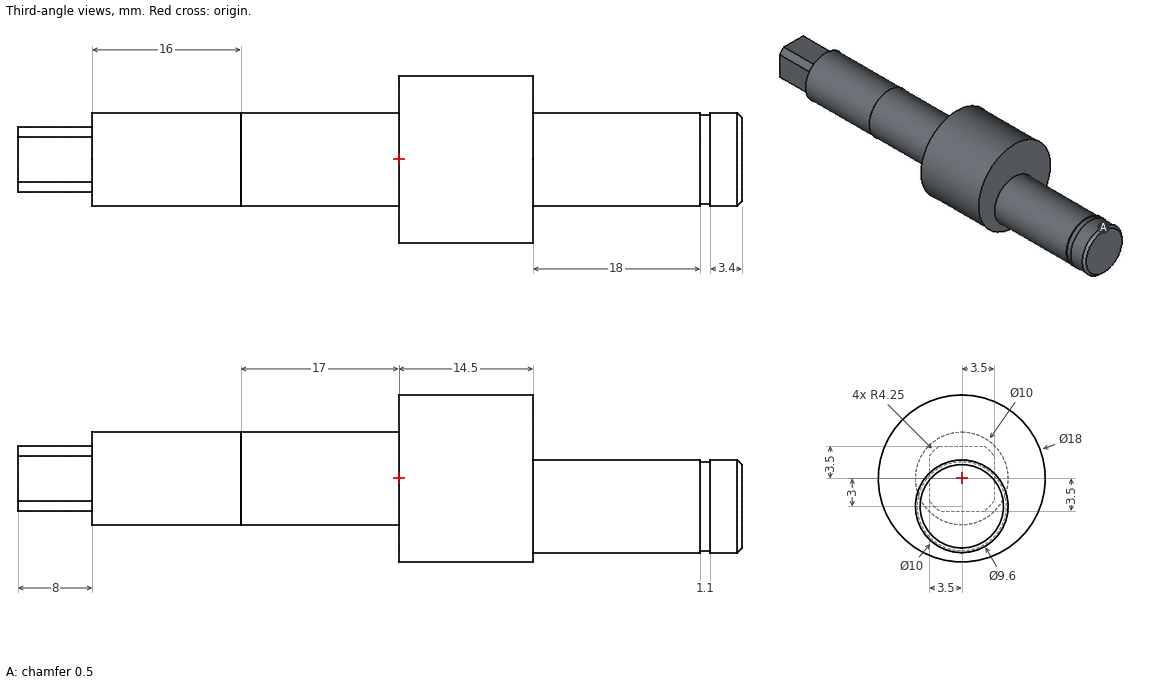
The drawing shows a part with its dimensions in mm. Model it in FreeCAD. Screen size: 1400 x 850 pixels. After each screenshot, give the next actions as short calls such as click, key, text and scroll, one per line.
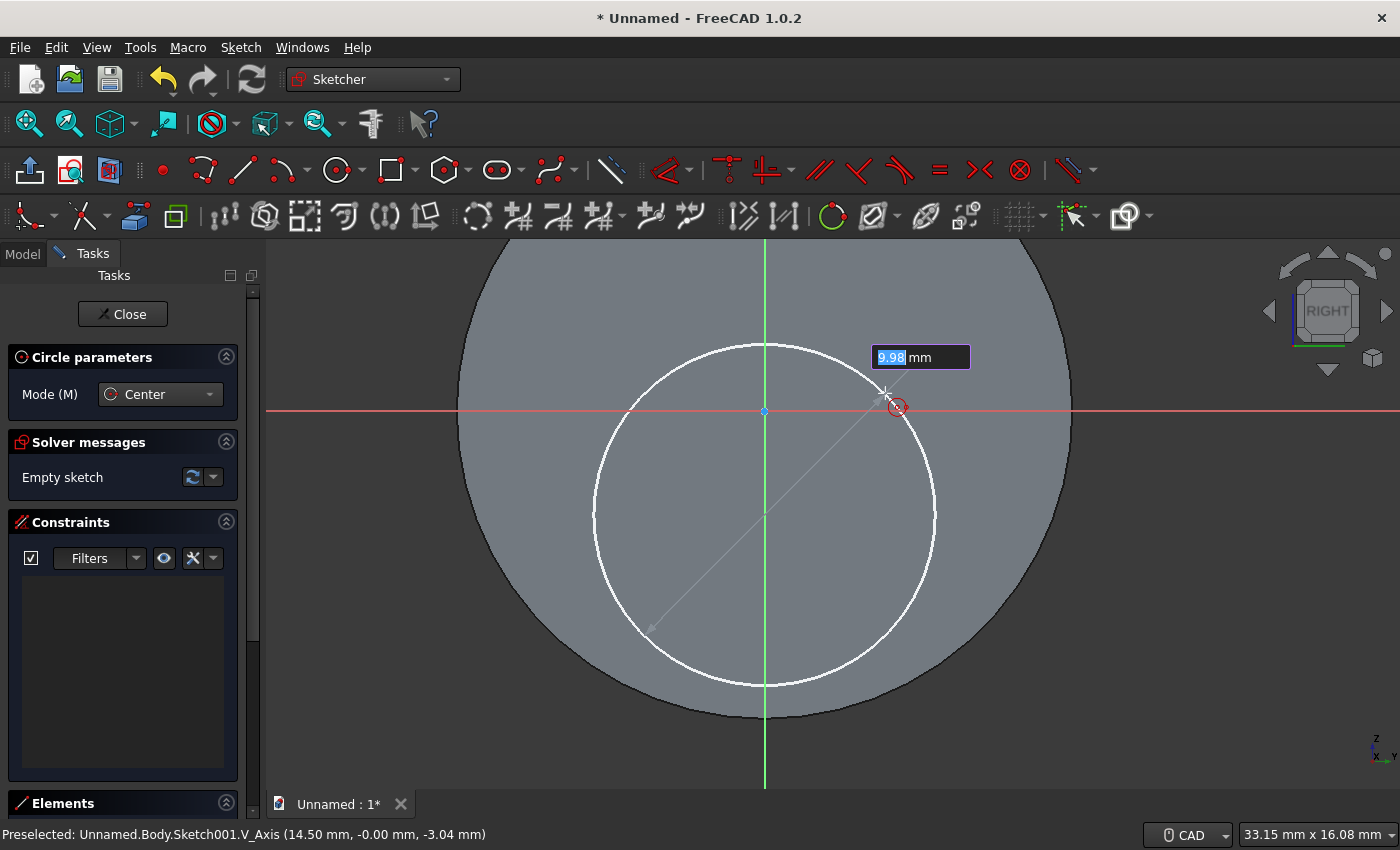
text(10)
key(Return)
key(Escape)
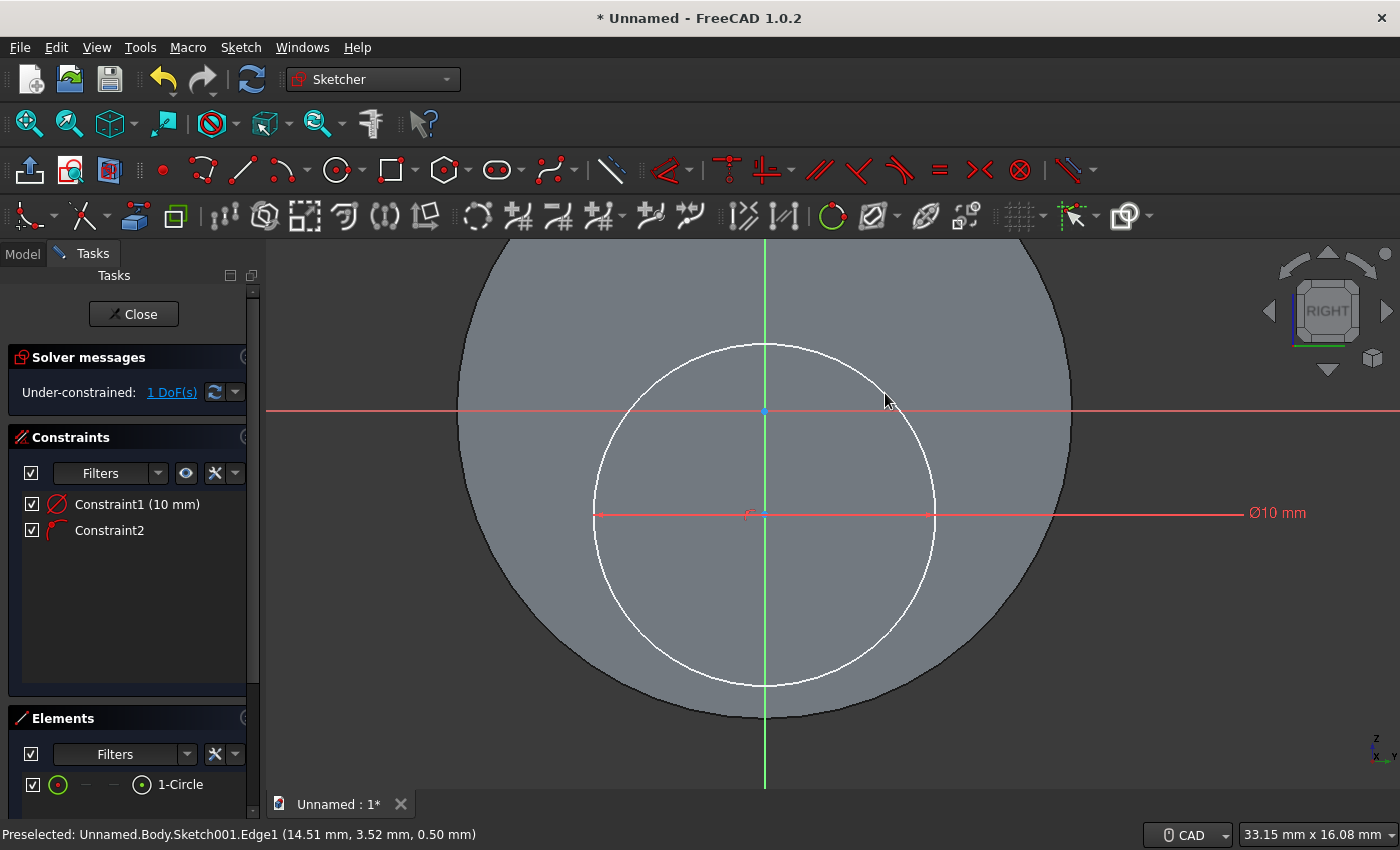
click(666, 170)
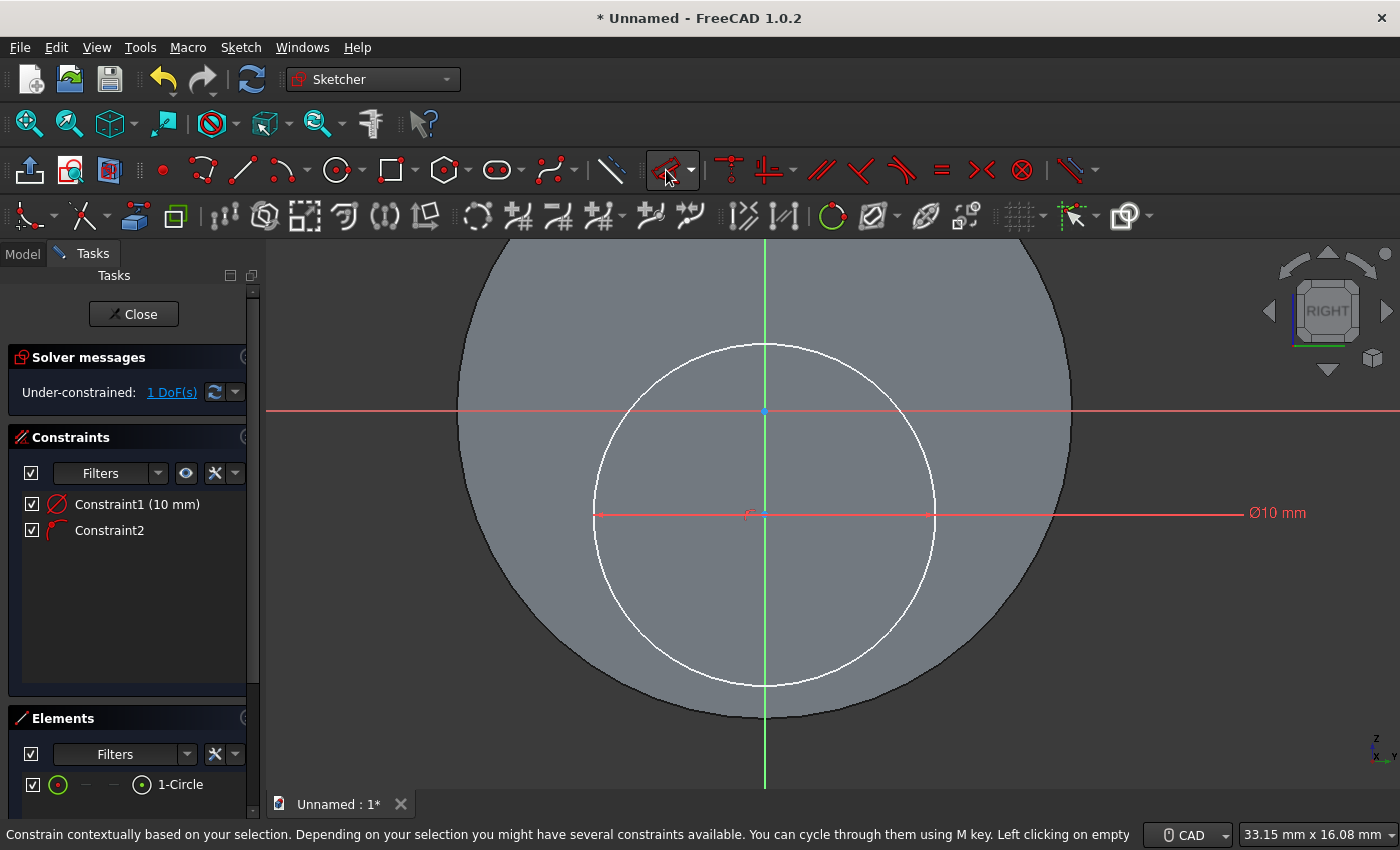
click(765, 515)
click(799, 463)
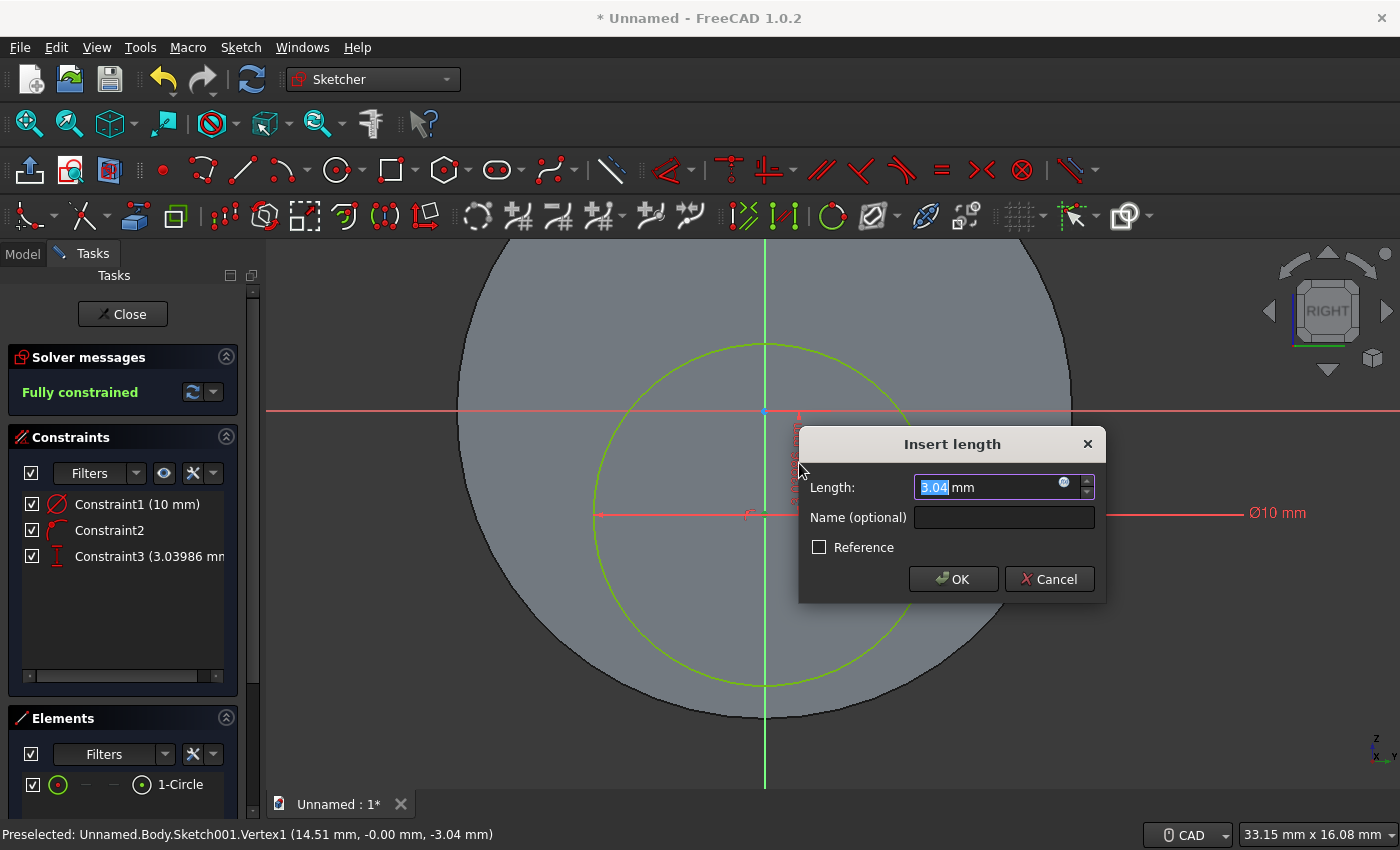
text(3)
key(Return)
key(Escape)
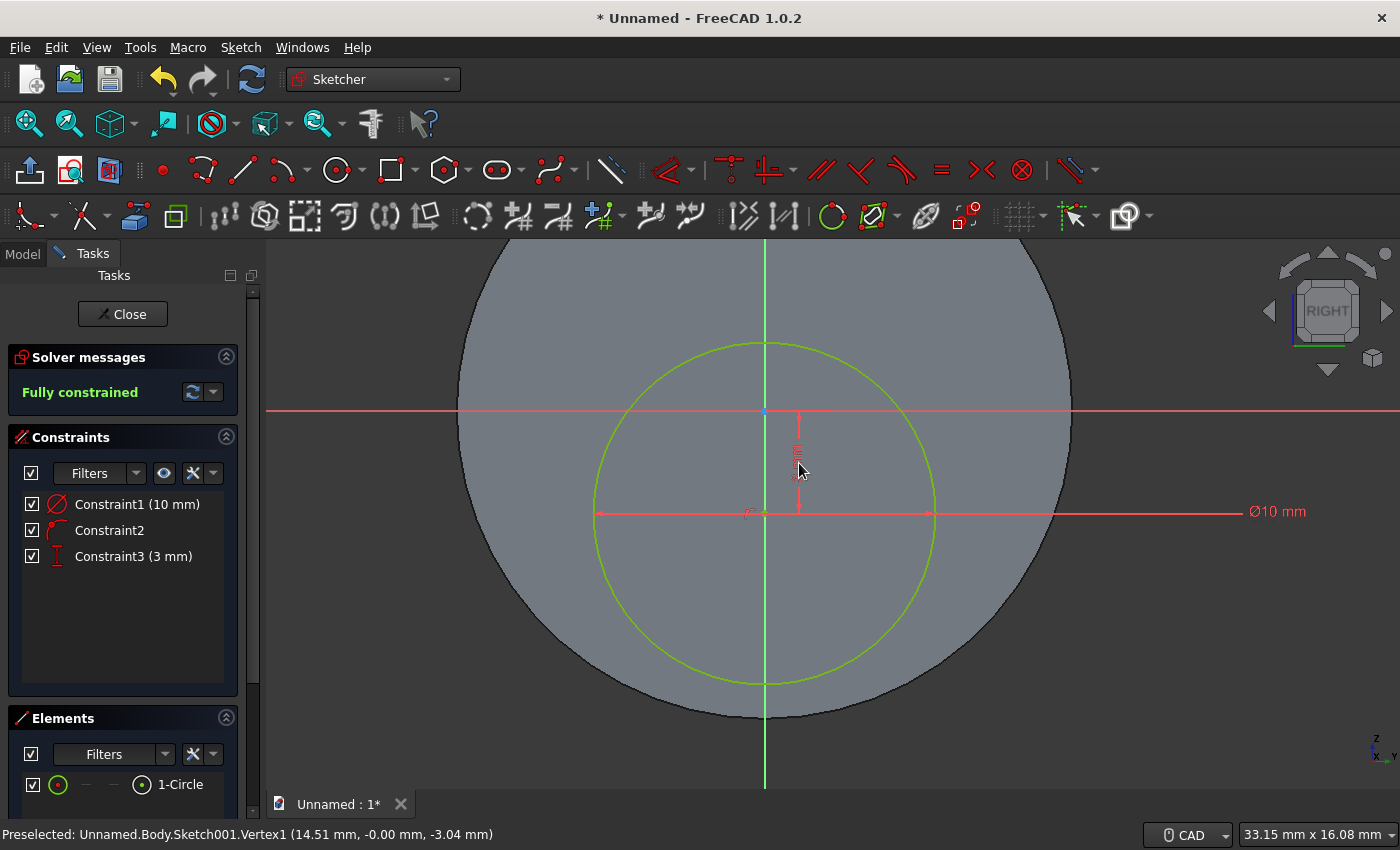
click(123, 314)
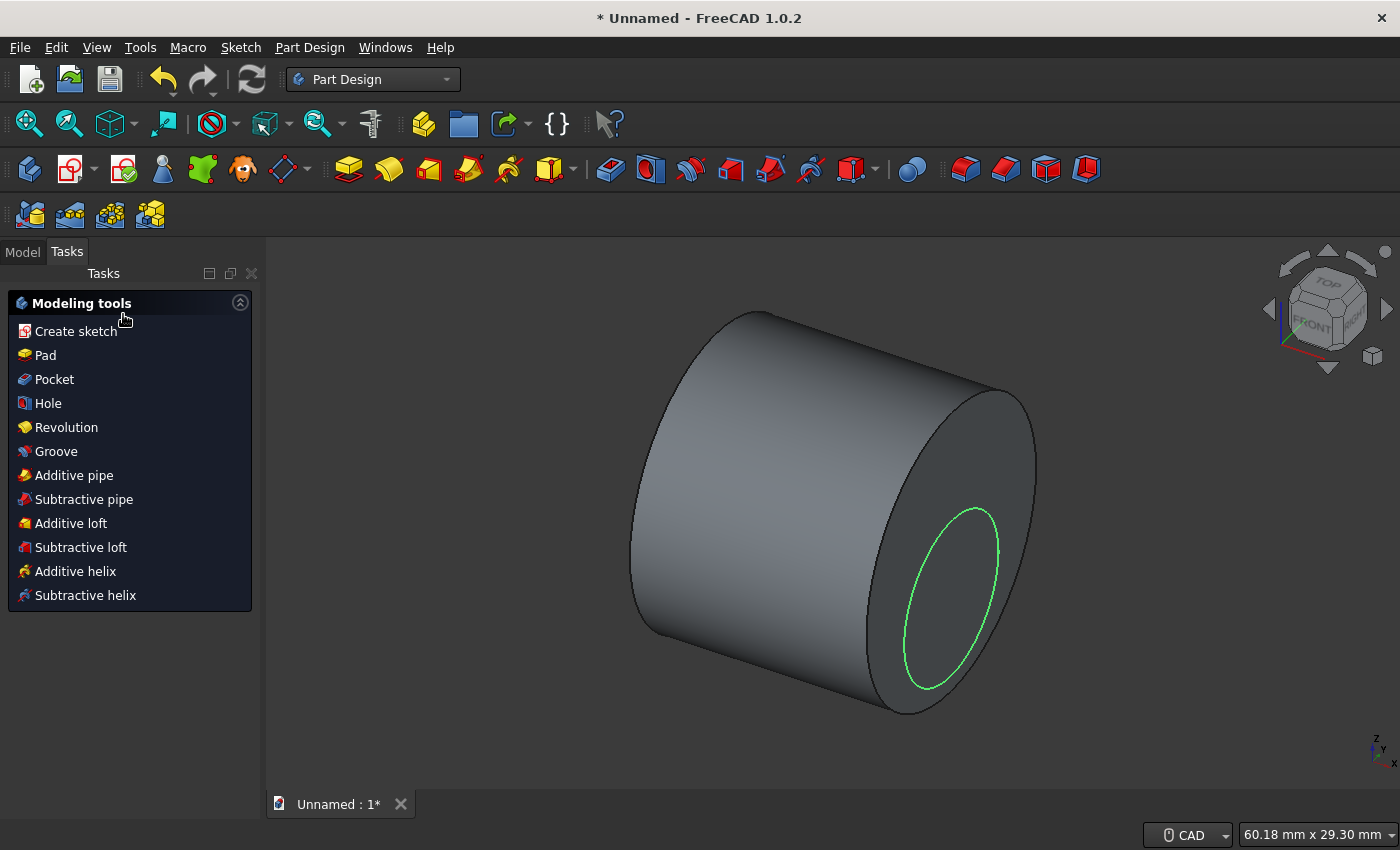
click(350, 170)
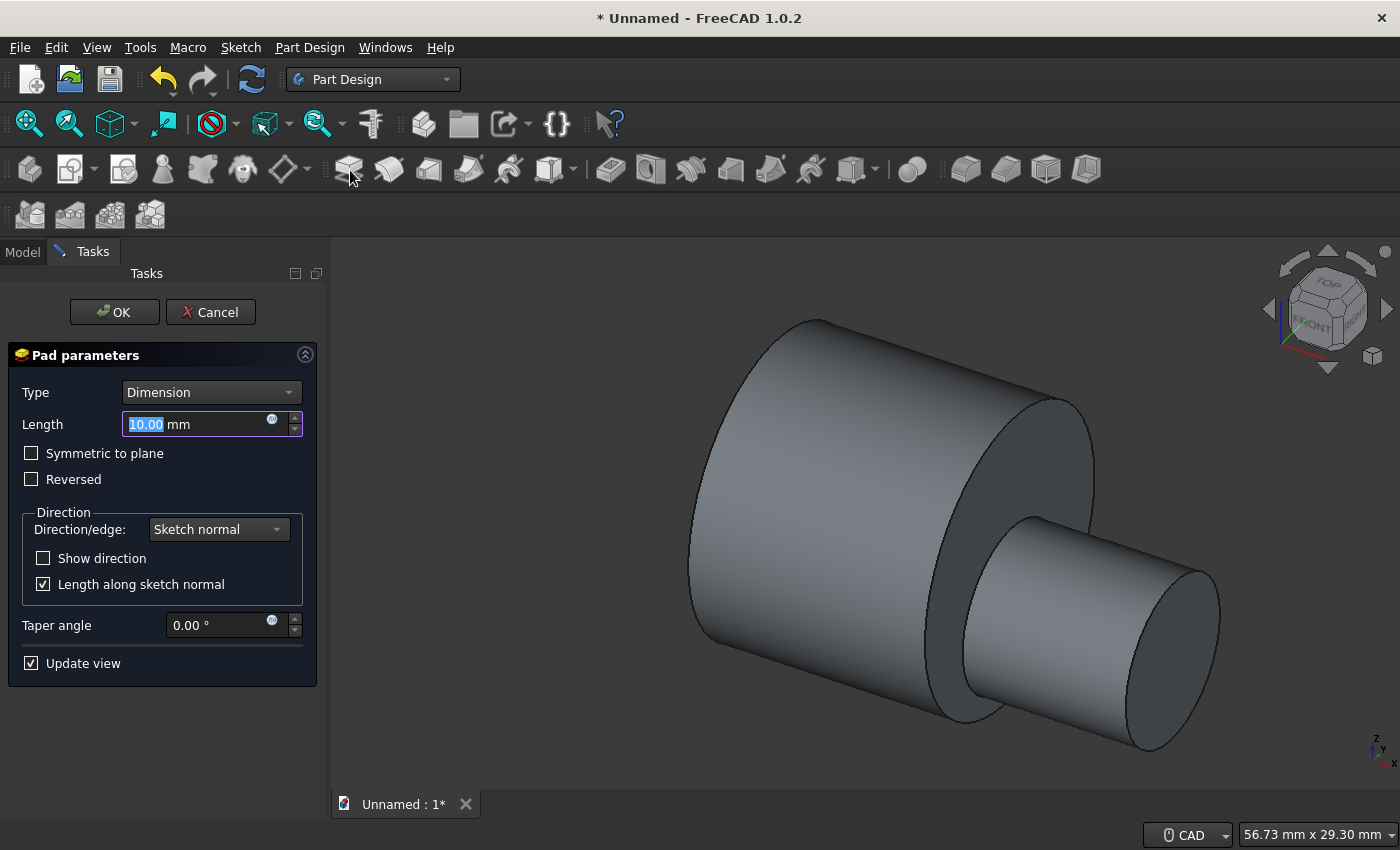
text(18)
key(Tab)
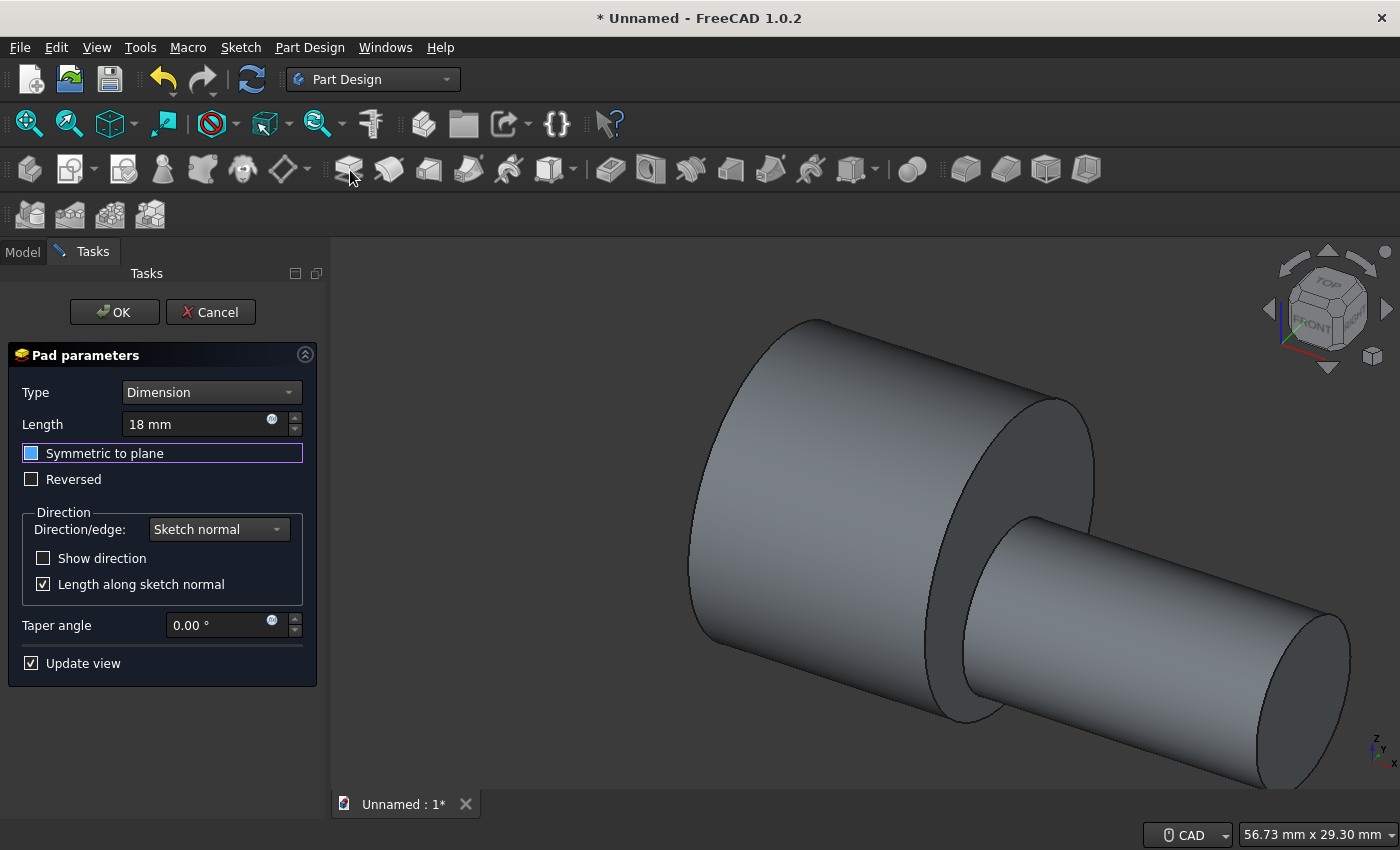
click(115, 312)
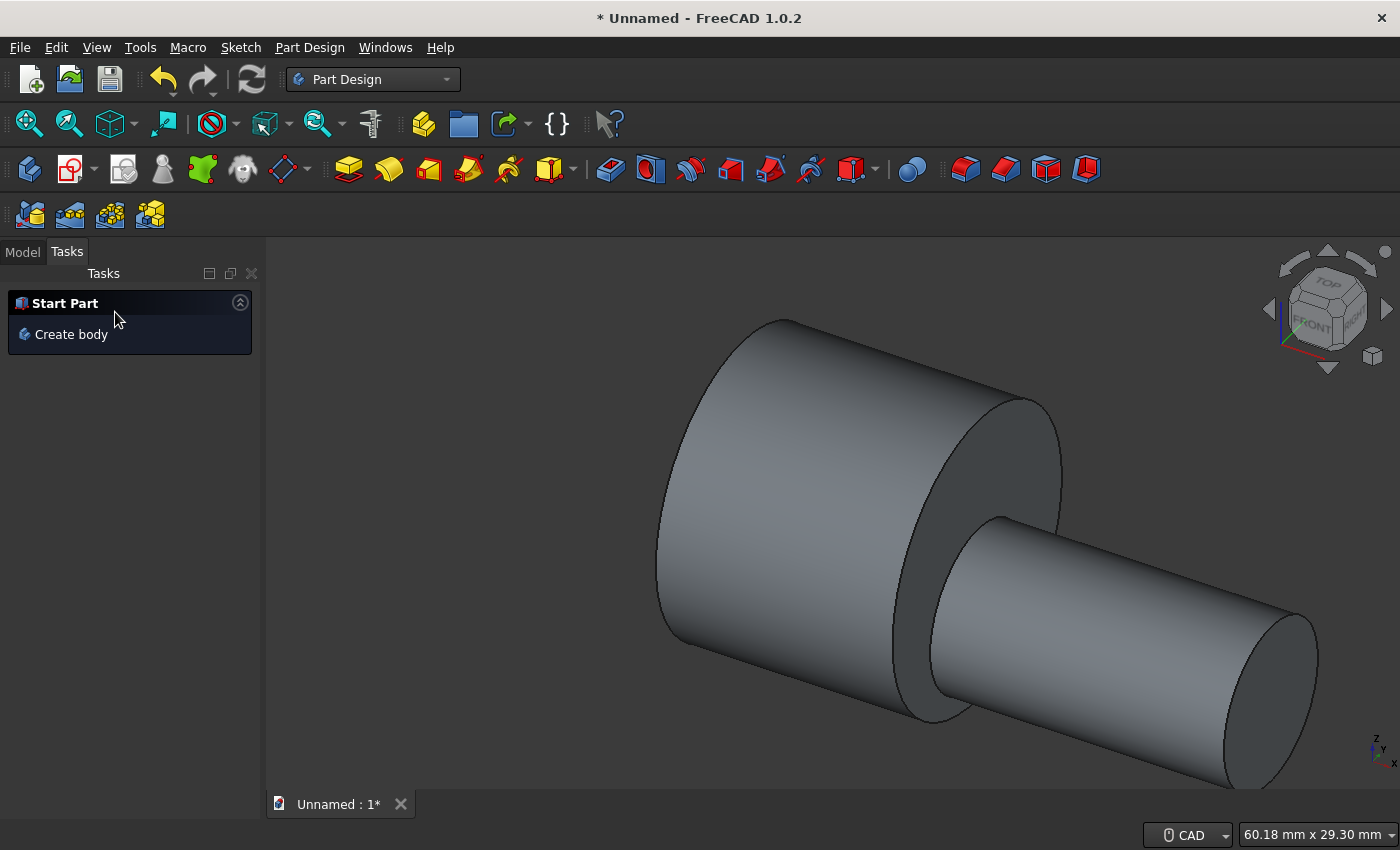
click(30, 124)